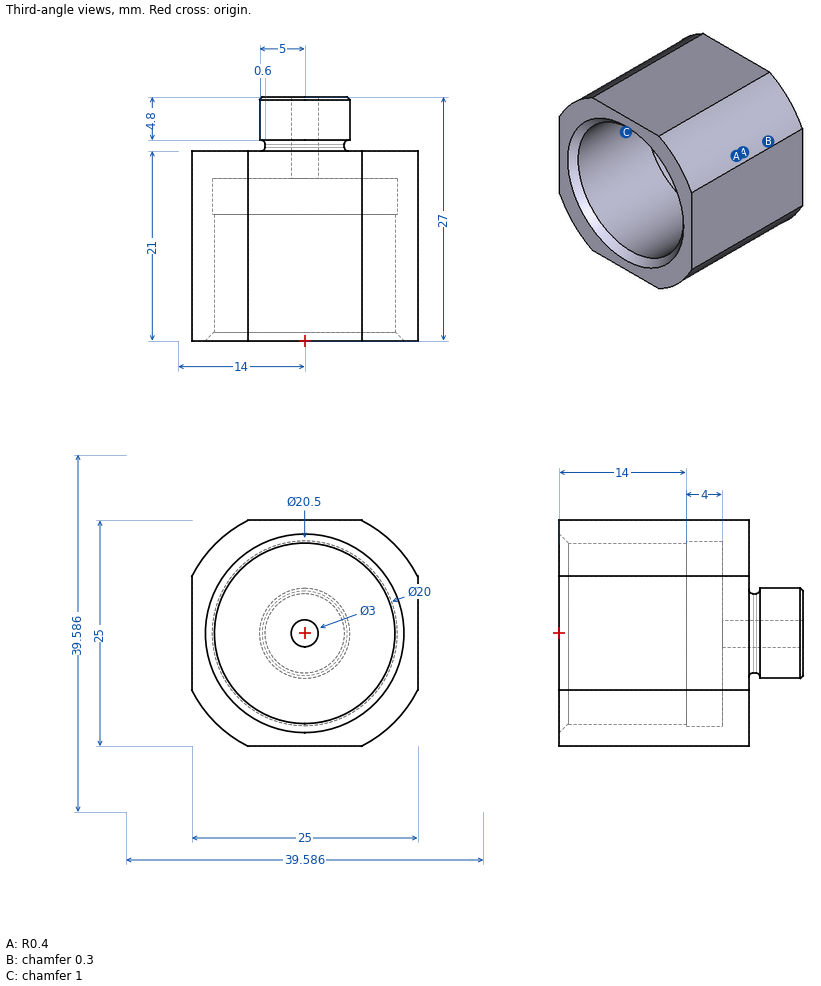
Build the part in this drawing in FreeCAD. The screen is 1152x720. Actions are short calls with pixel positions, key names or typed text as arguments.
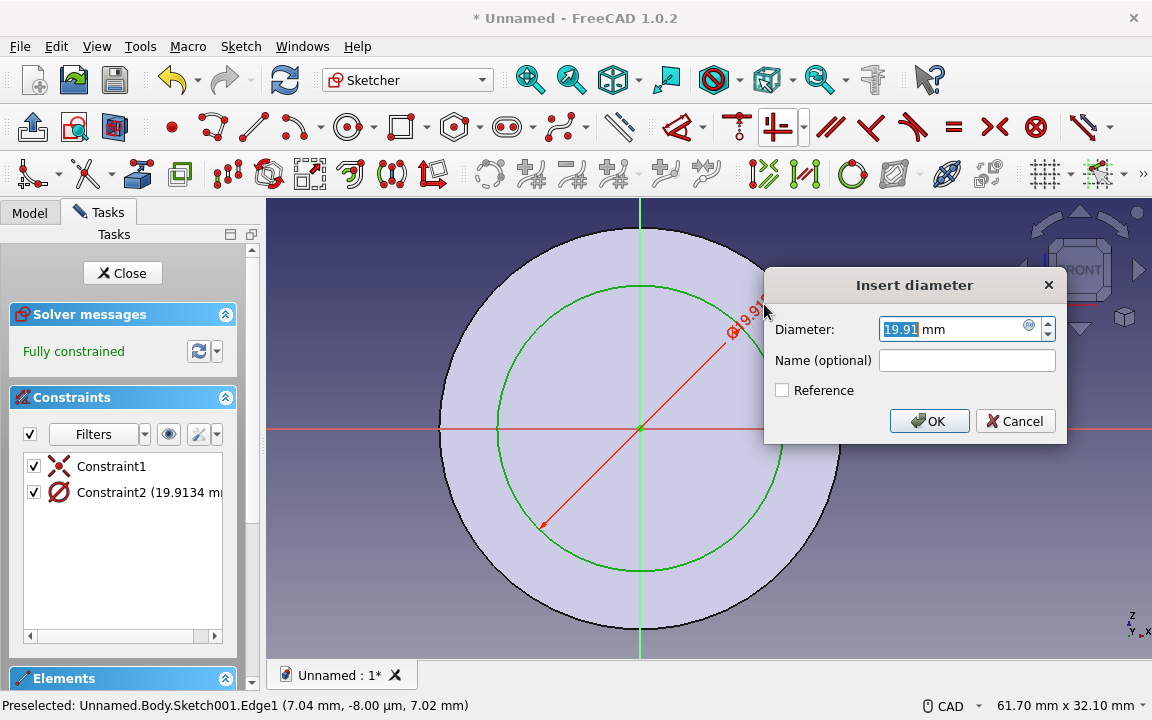
text(20)
key(Return)
key(Escape)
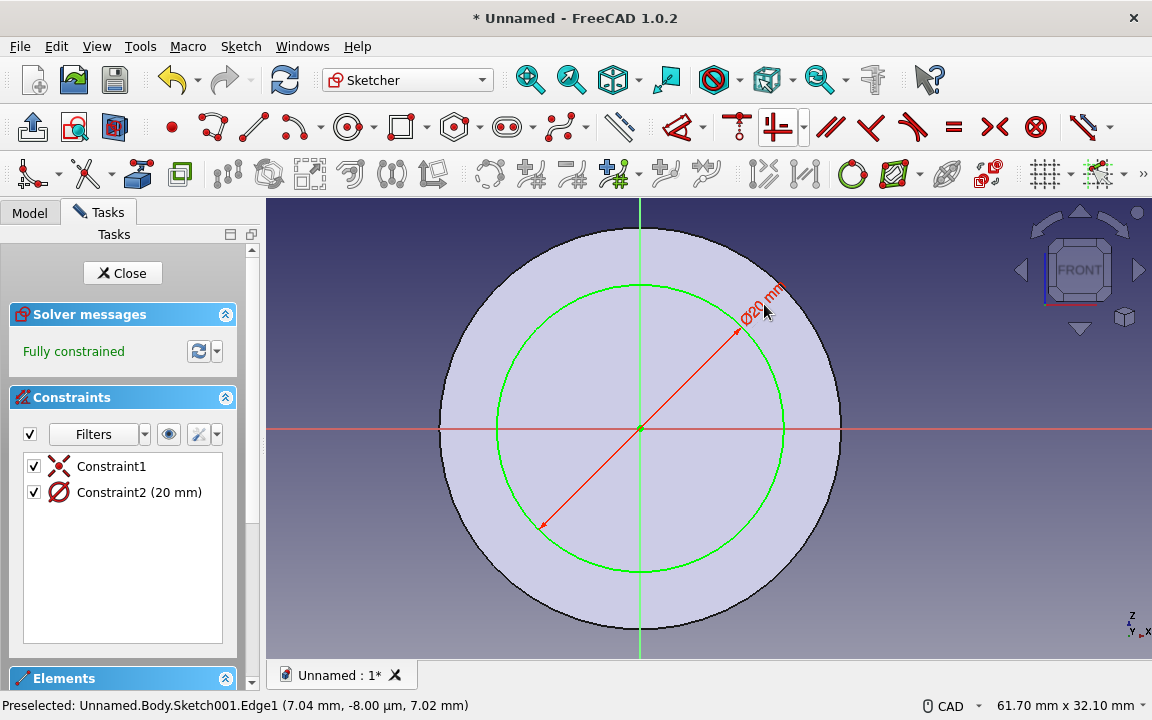
click(123, 273)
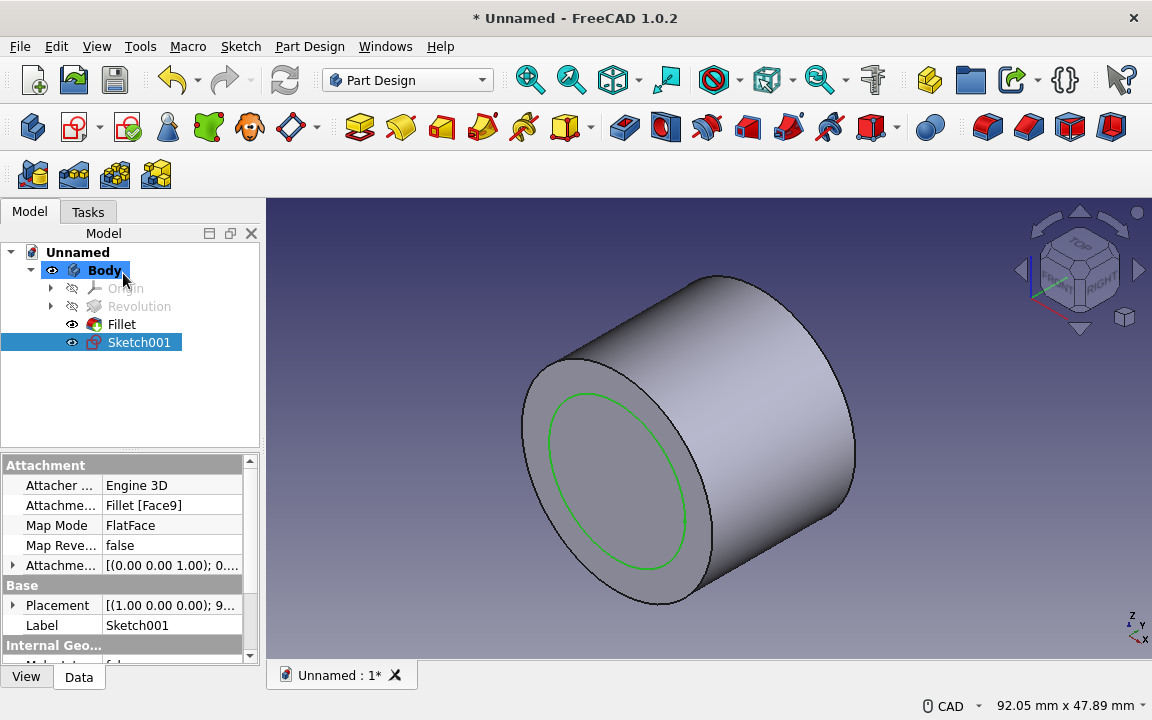
click(625, 128)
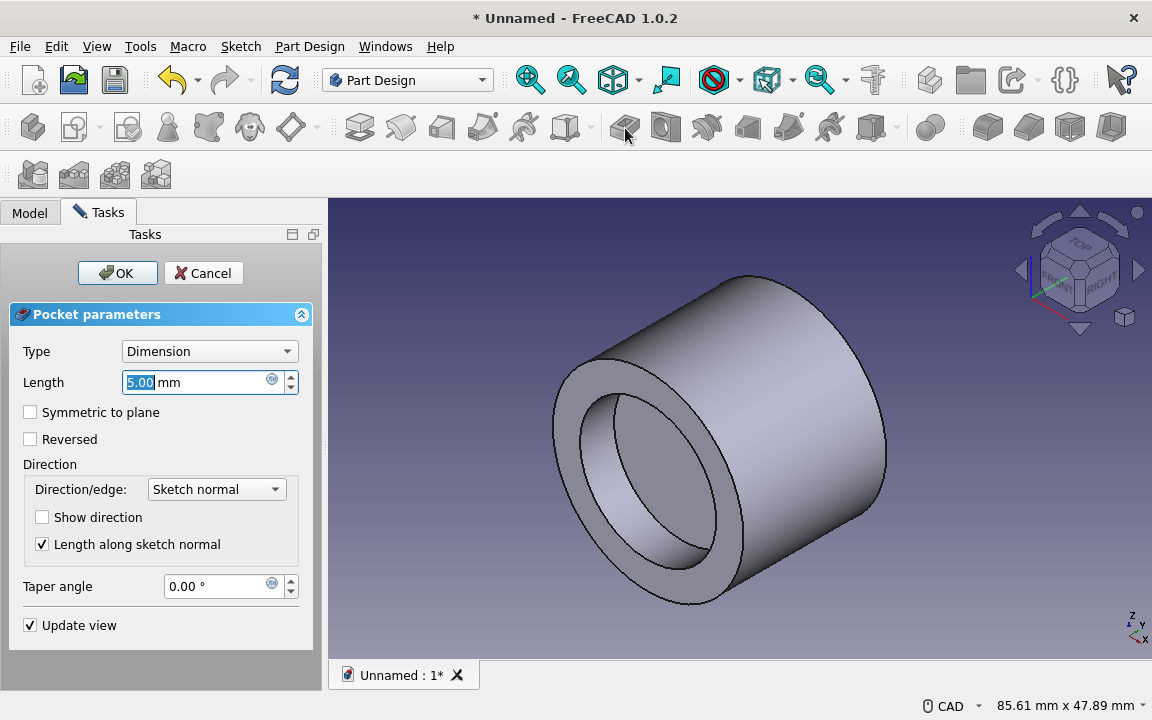
text(14)
key(Tab)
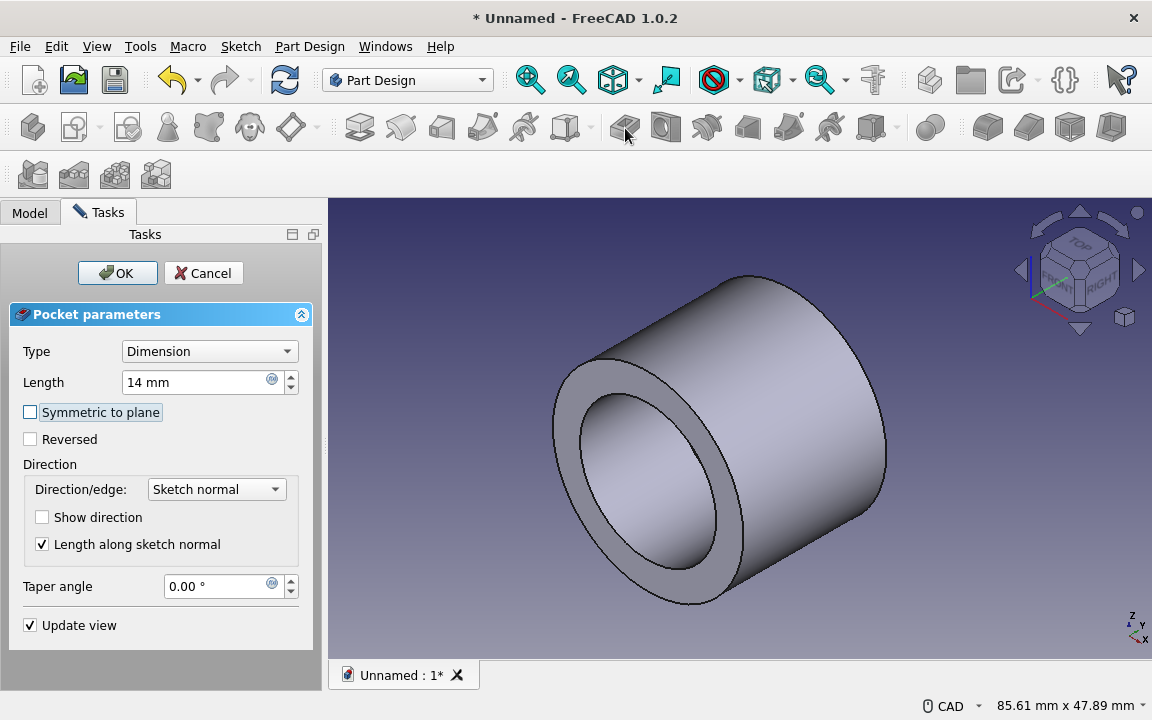
click(118, 273)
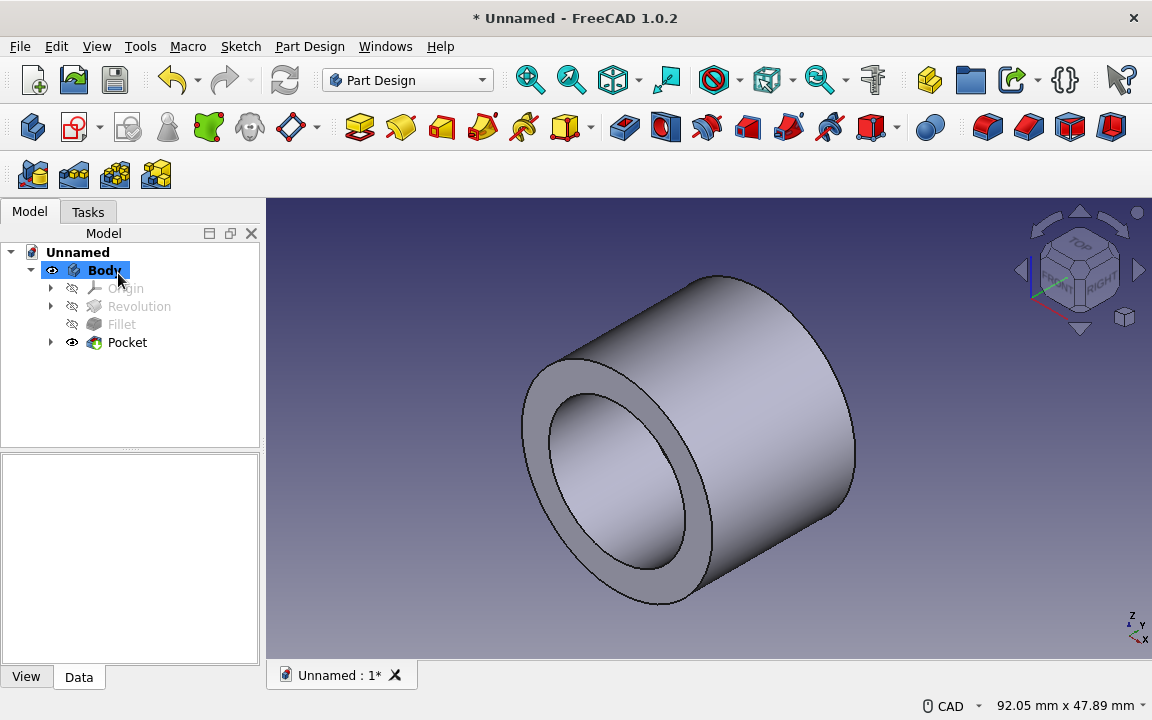
key(1)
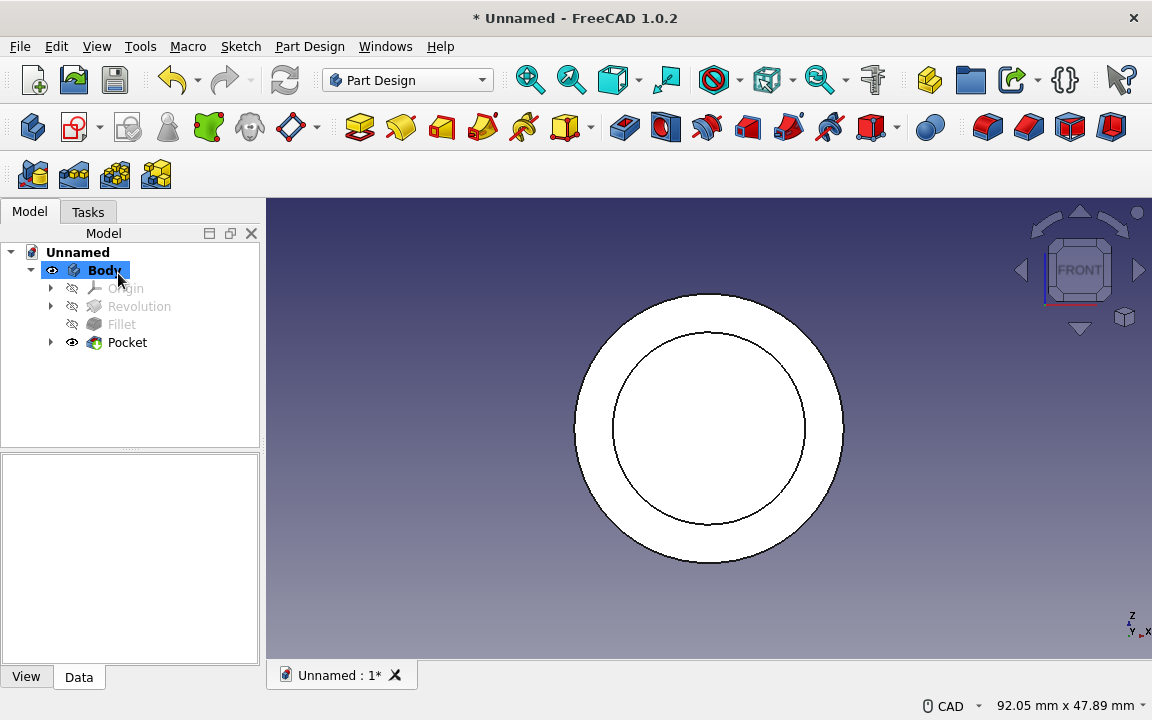
click(709, 427)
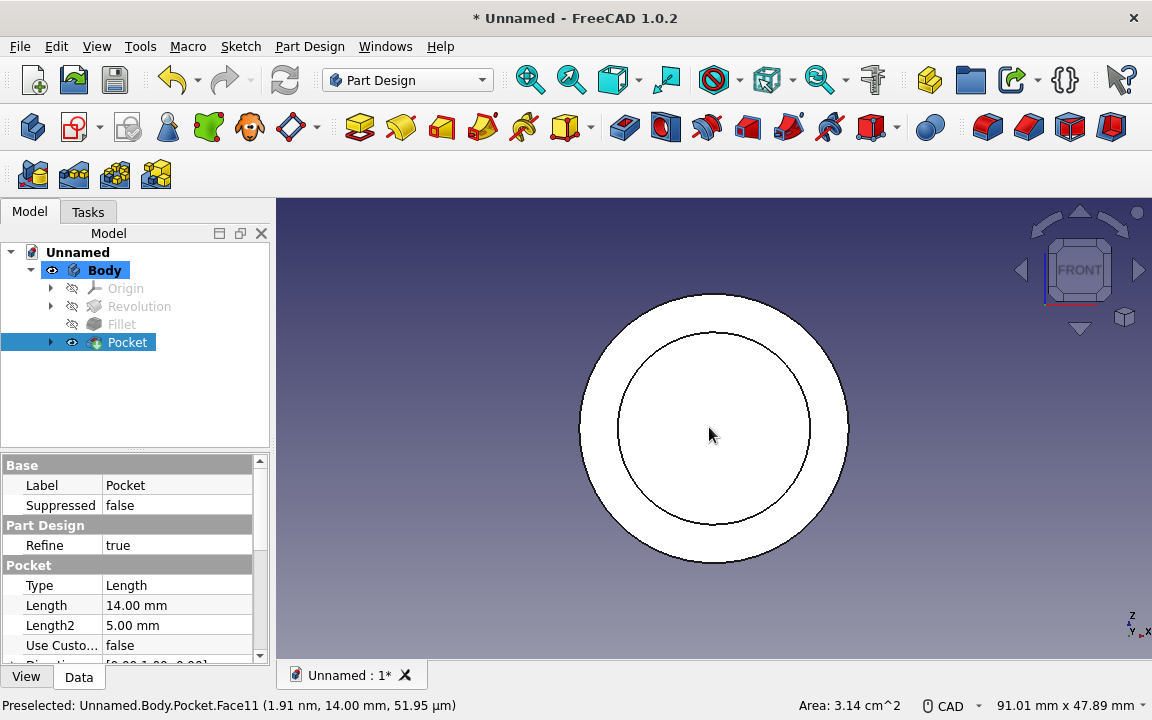
click(74, 128)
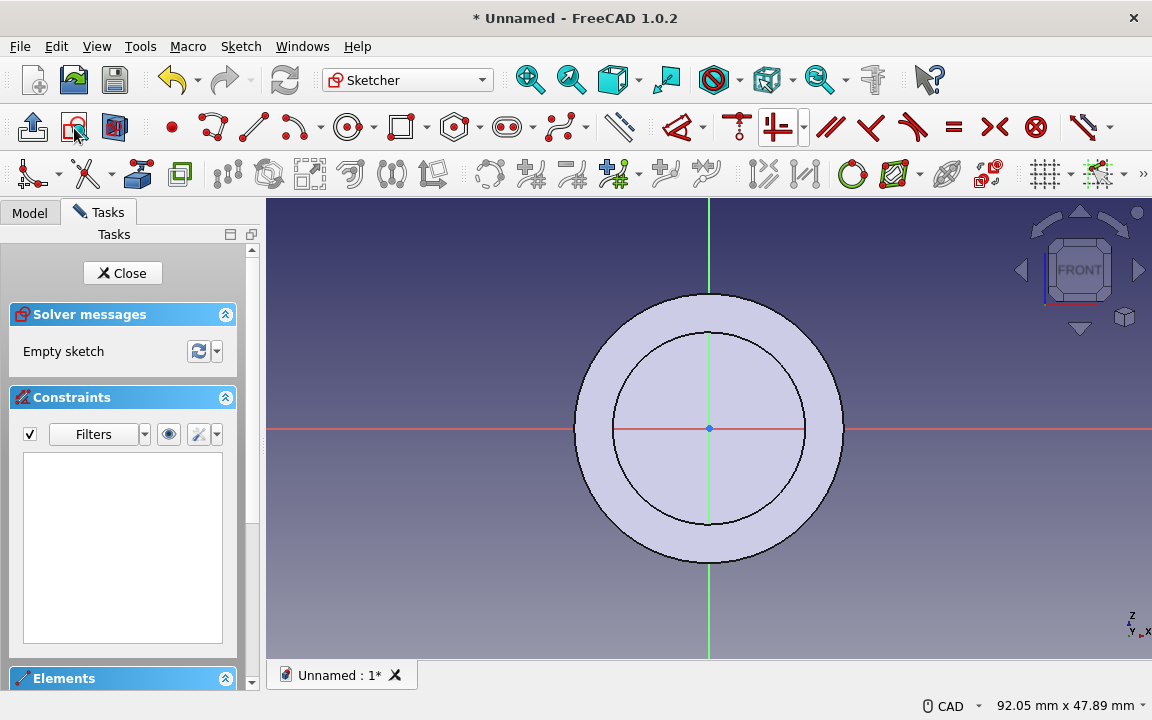
click(115, 128)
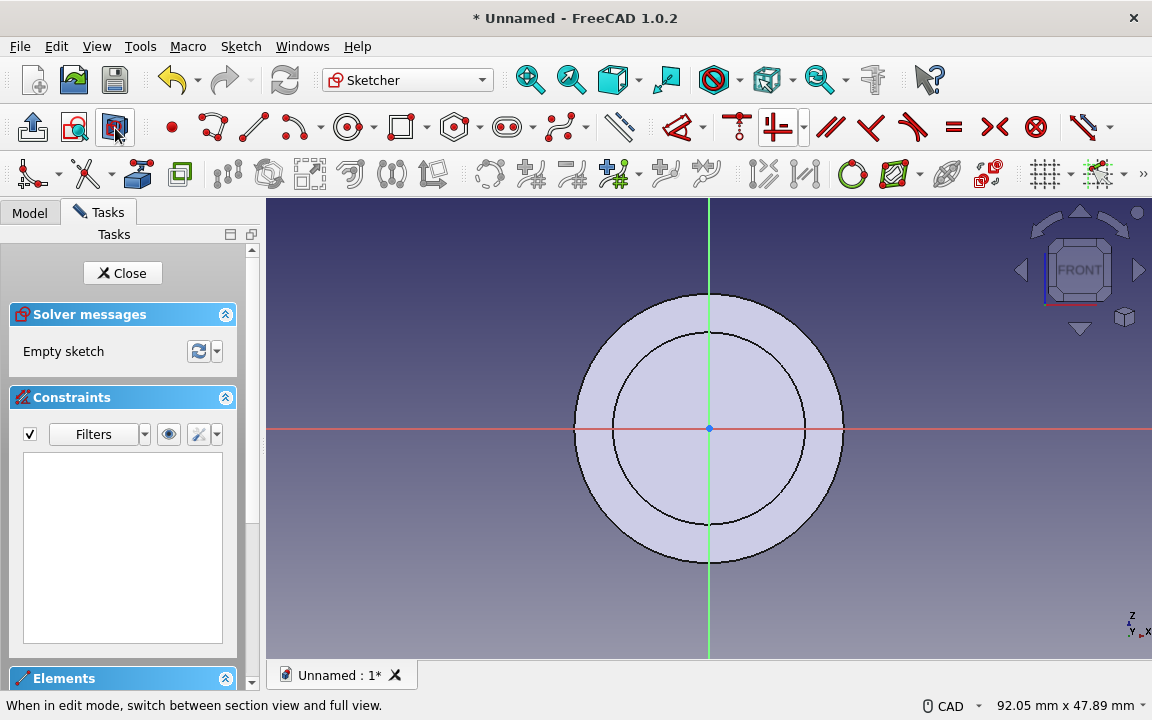
scroll(848, 428, up, 2)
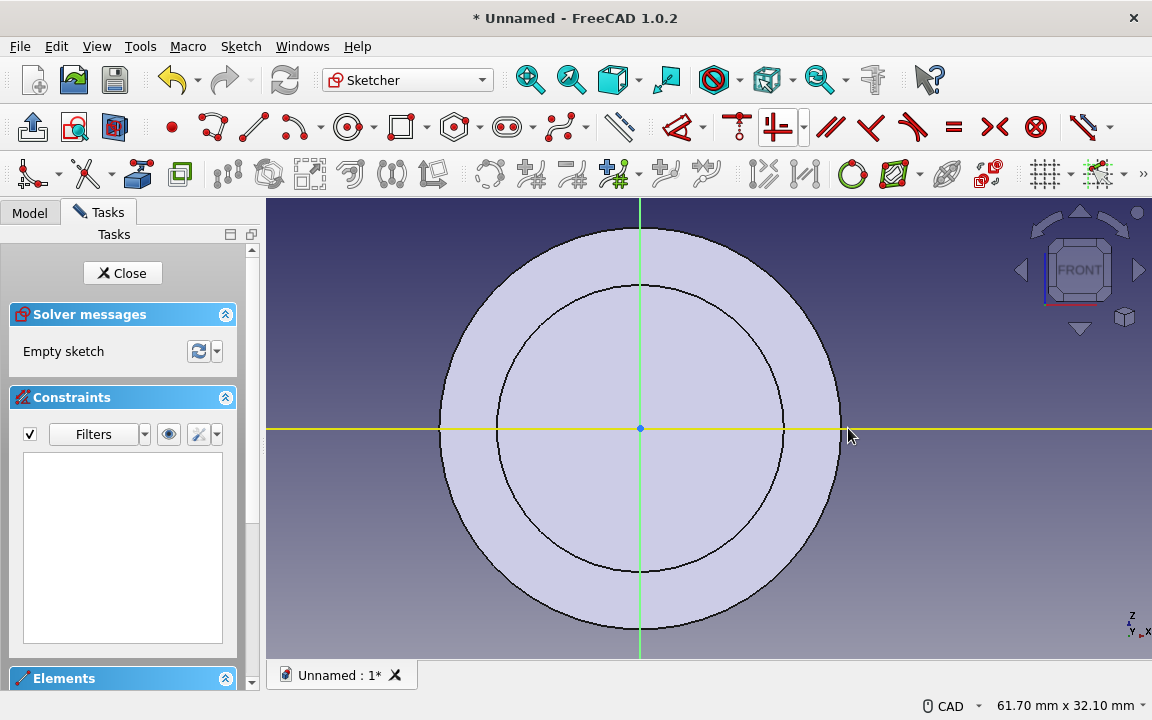
click(348, 128)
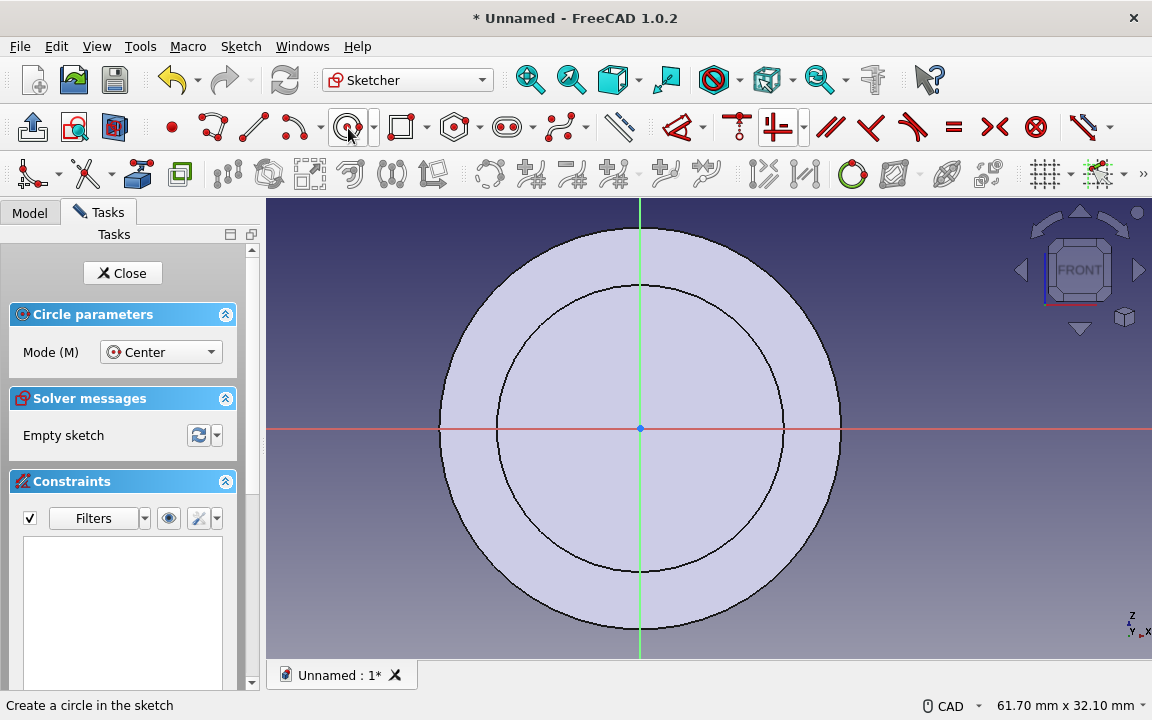
click(640, 428)
click(744, 324)
key(Escape)